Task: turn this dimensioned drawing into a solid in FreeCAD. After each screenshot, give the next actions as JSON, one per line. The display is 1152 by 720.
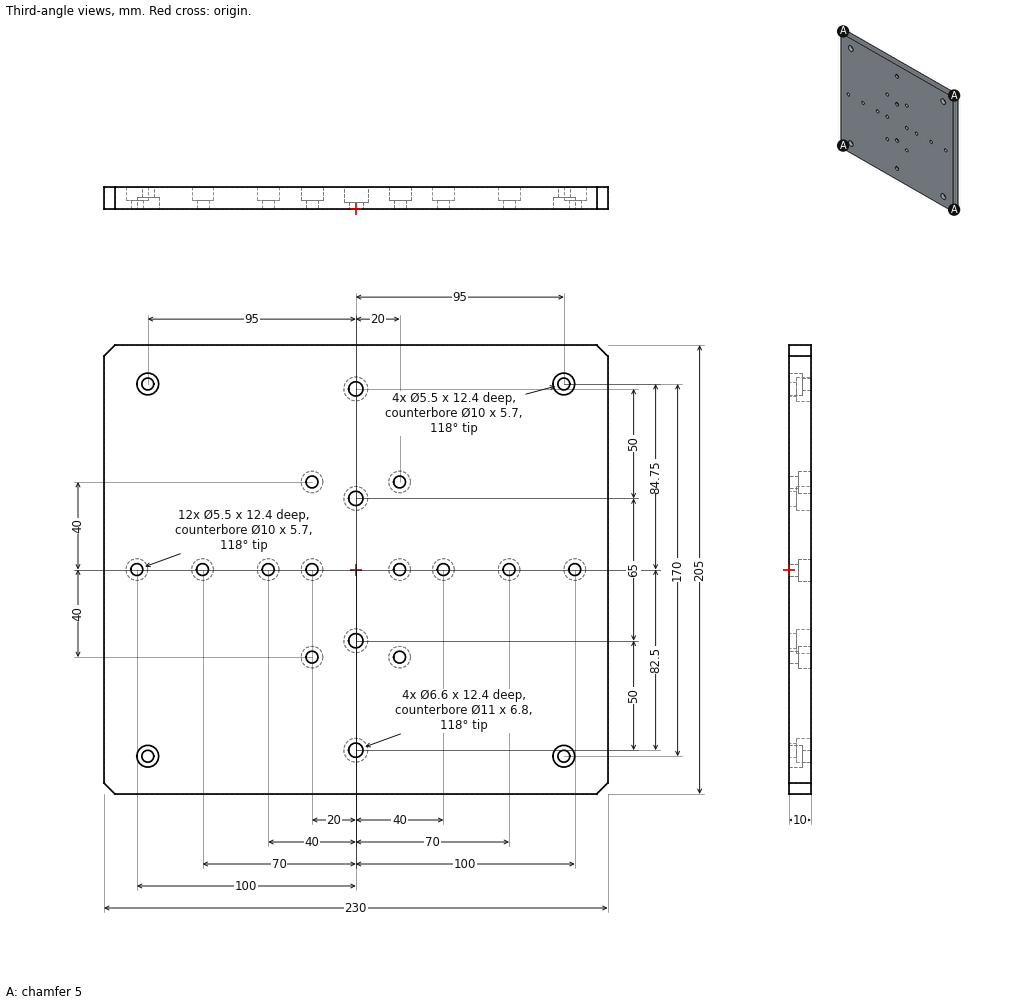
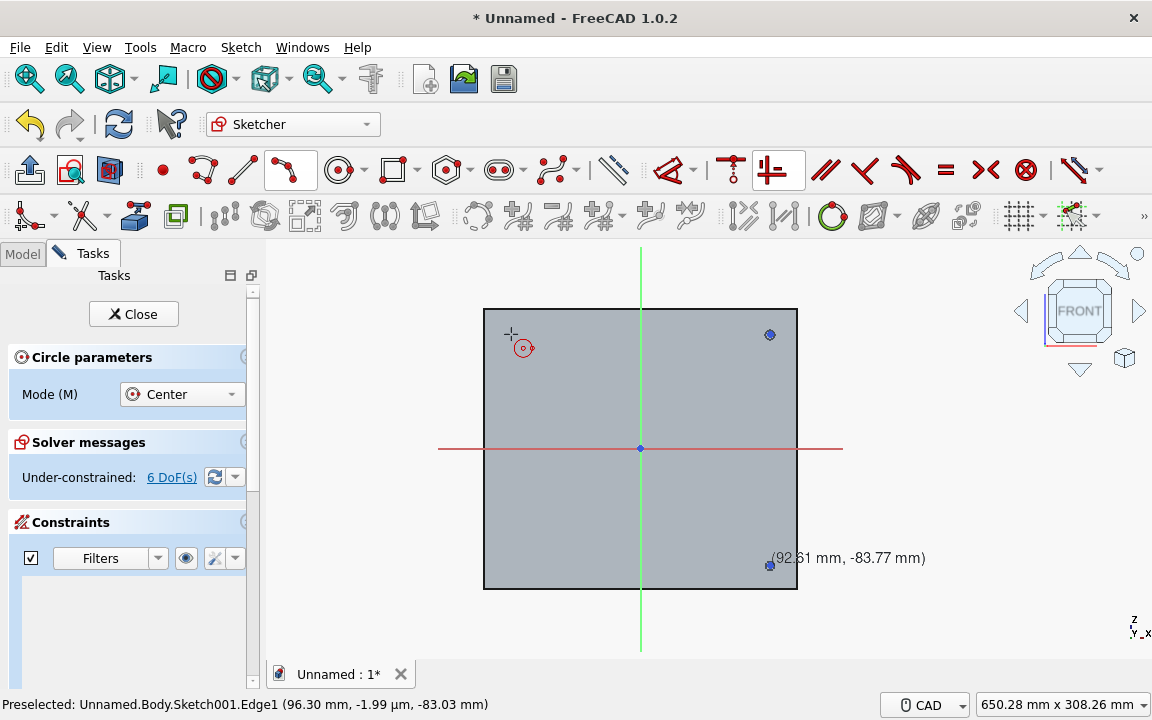
{"action": "left_click", "coordinate": [511, 334]}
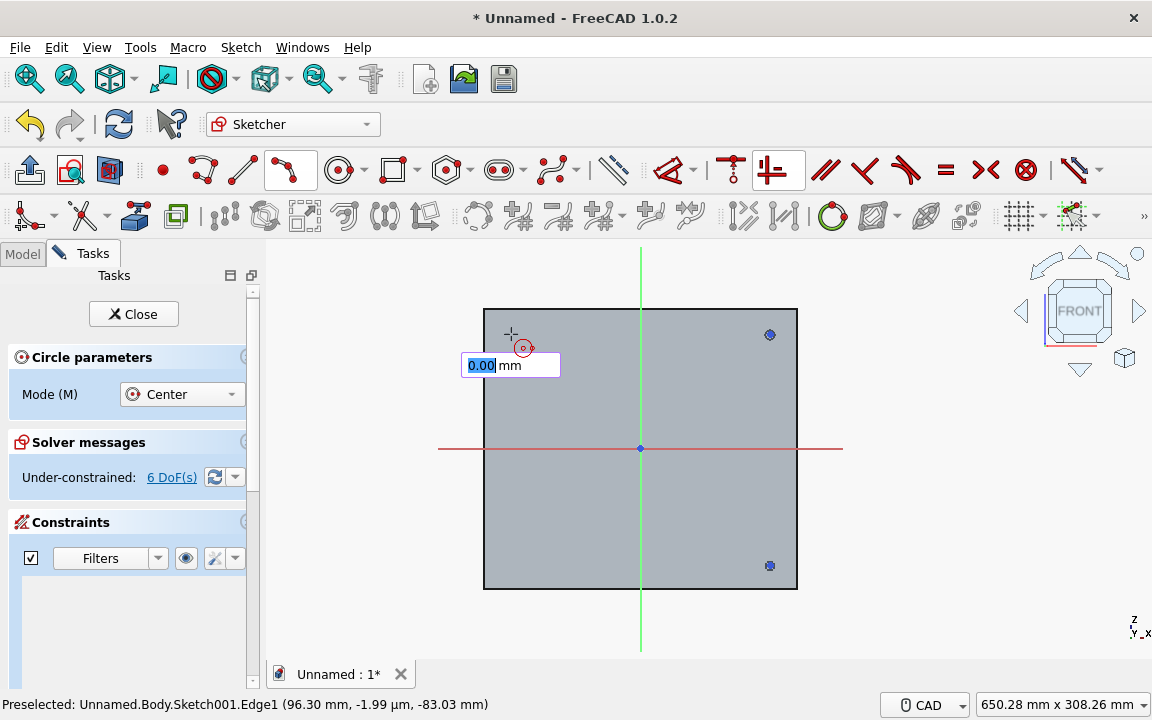
{"action": "scroll", "coordinate": [514, 331], "scroll_direction": "up", "scroll_amount": 8}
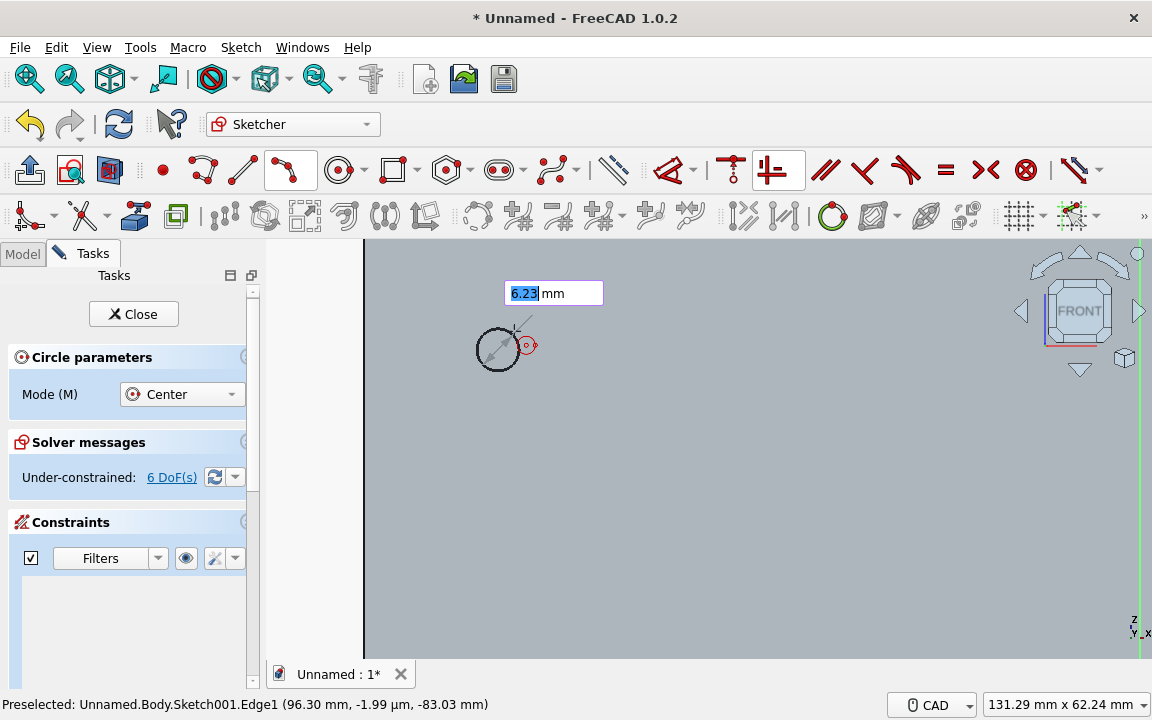
{"action": "left_click", "coordinate": [512, 330]}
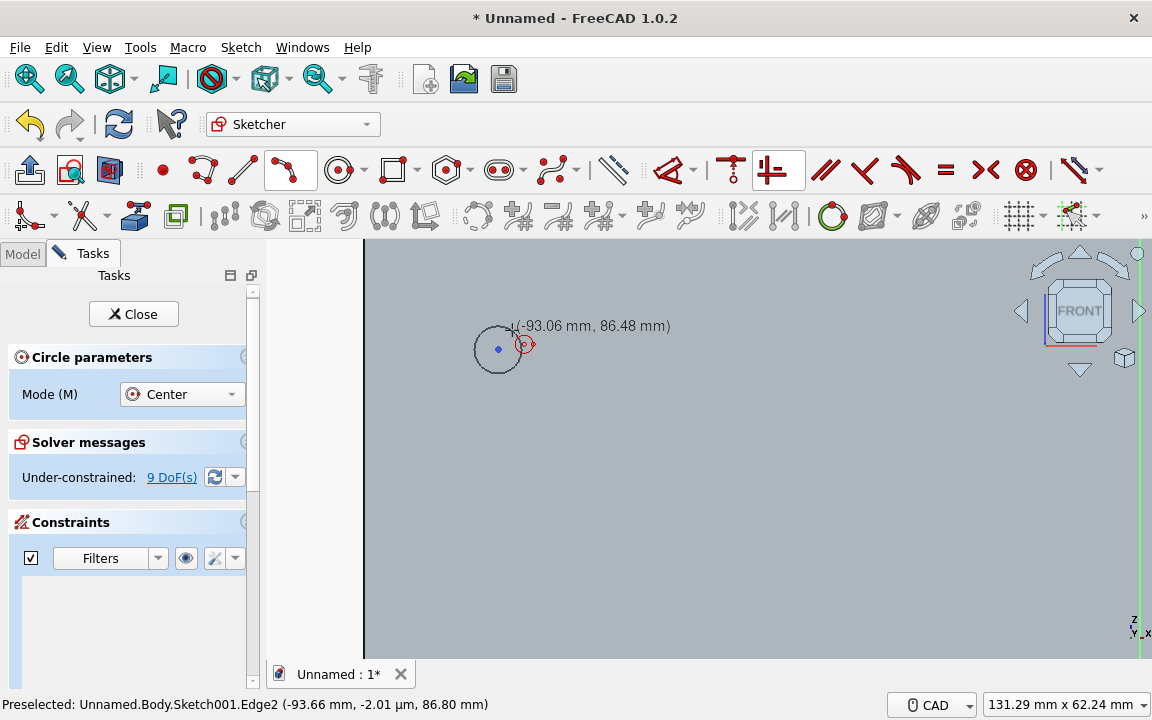
{"action": "scroll", "coordinate": [514, 331], "scroll_direction": "down", "scroll_amount": 8}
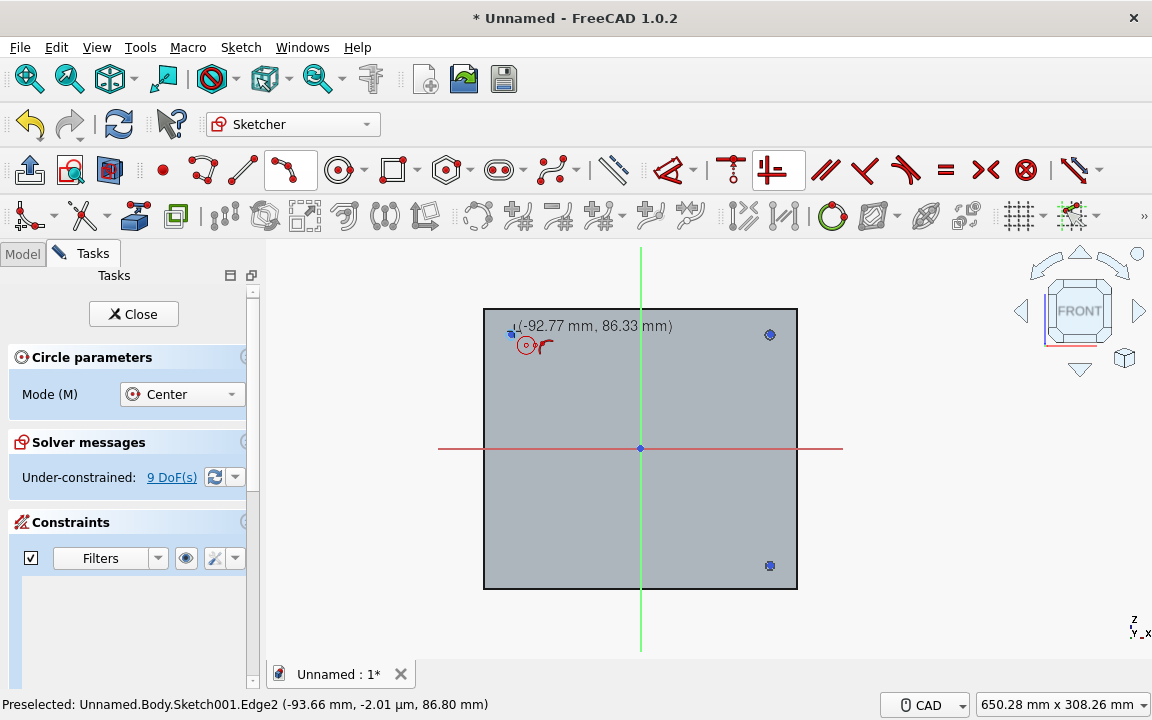
{"action": "scroll", "coordinate": [511, 565], "scroll_direction": "up", "scroll_amount": 10}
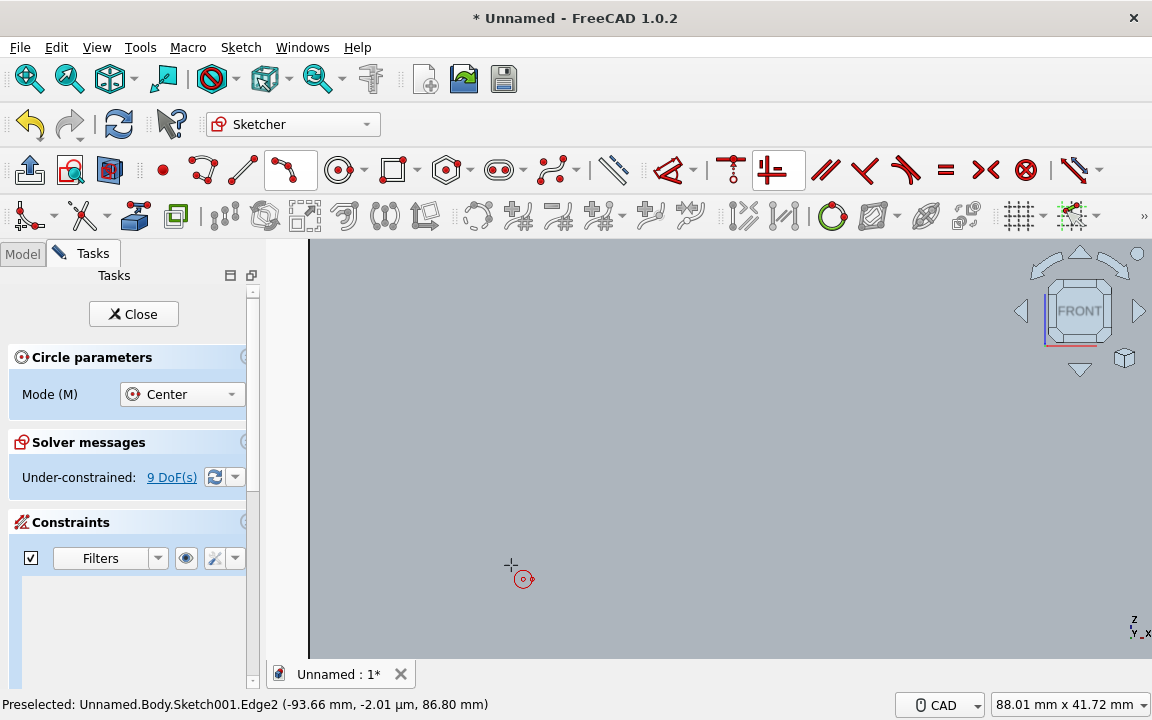
{"action": "scroll", "coordinate": [511, 565], "scroll_direction": "down", "scroll_amount": 10}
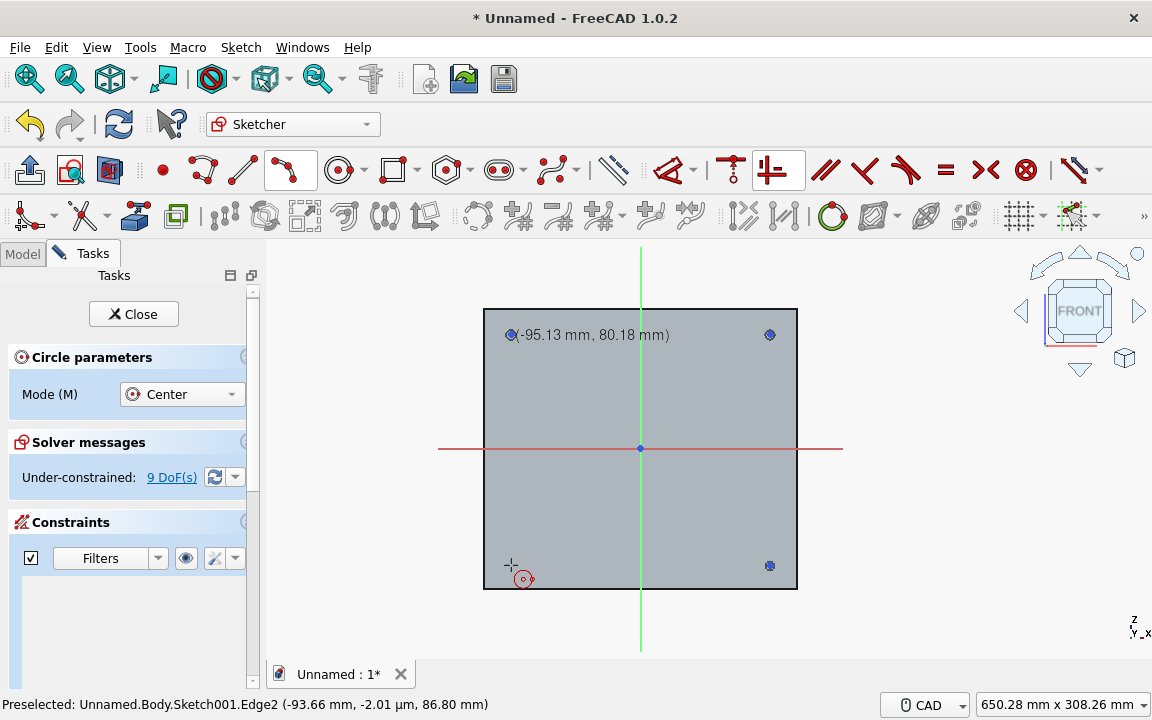
{"action": "left_click", "coordinate": [511, 565]}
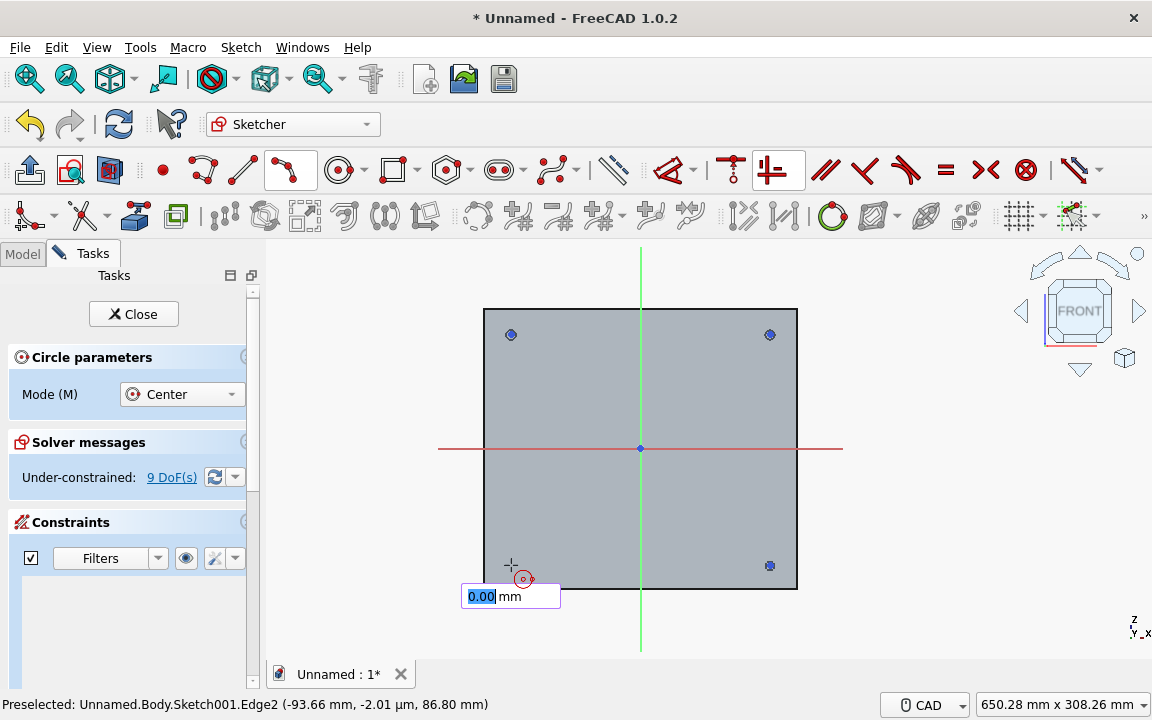
{"action": "scroll", "coordinate": [514, 563], "scroll_direction": "up", "scroll_amount": 8}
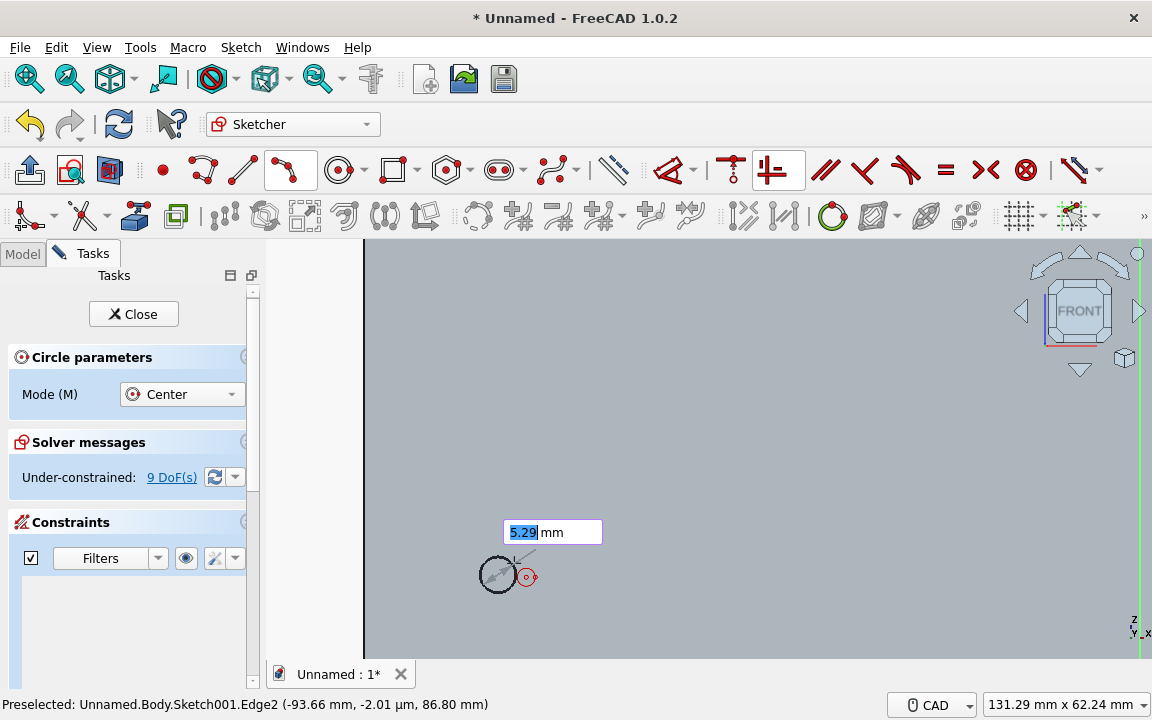
{"action": "left_click", "coordinate": [512, 557]}
{"action": "key", "text": "Escape"}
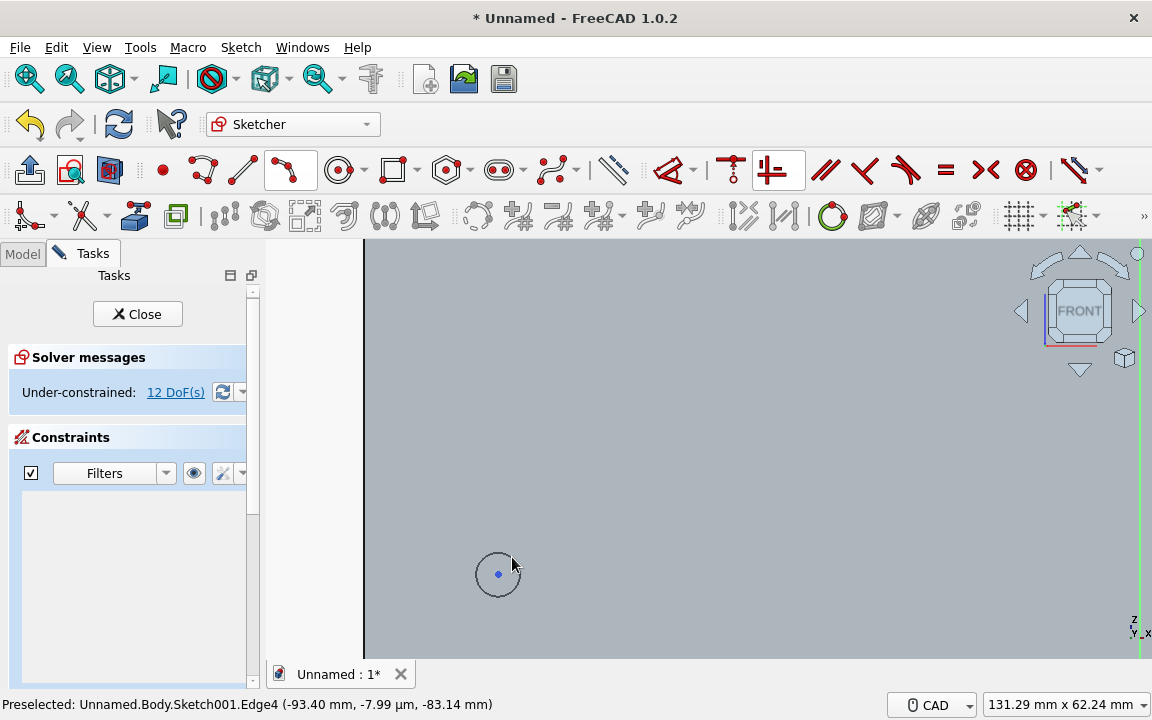
{"action": "scroll", "coordinate": [514, 563], "scroll_direction": "down", "scroll_amount": 8}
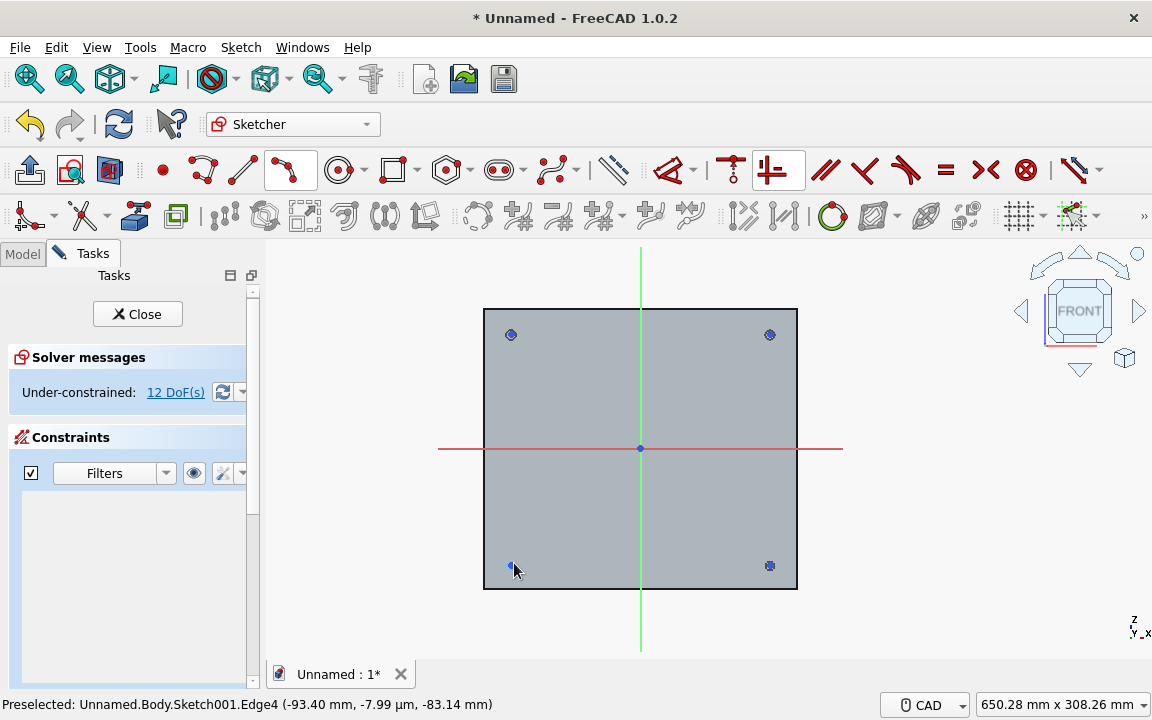
{"action": "scroll", "coordinate": [773, 332], "scroll_direction": "up", "scroll_amount": 6}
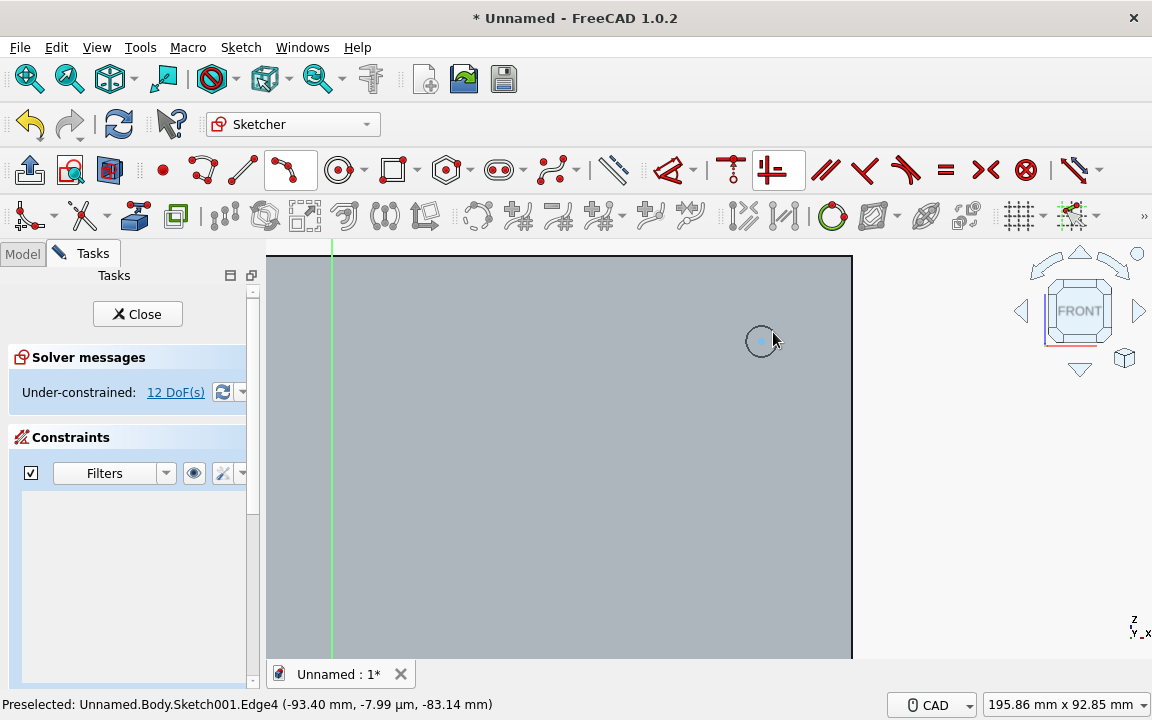
{"action": "left_click", "coordinate": [773, 330]}